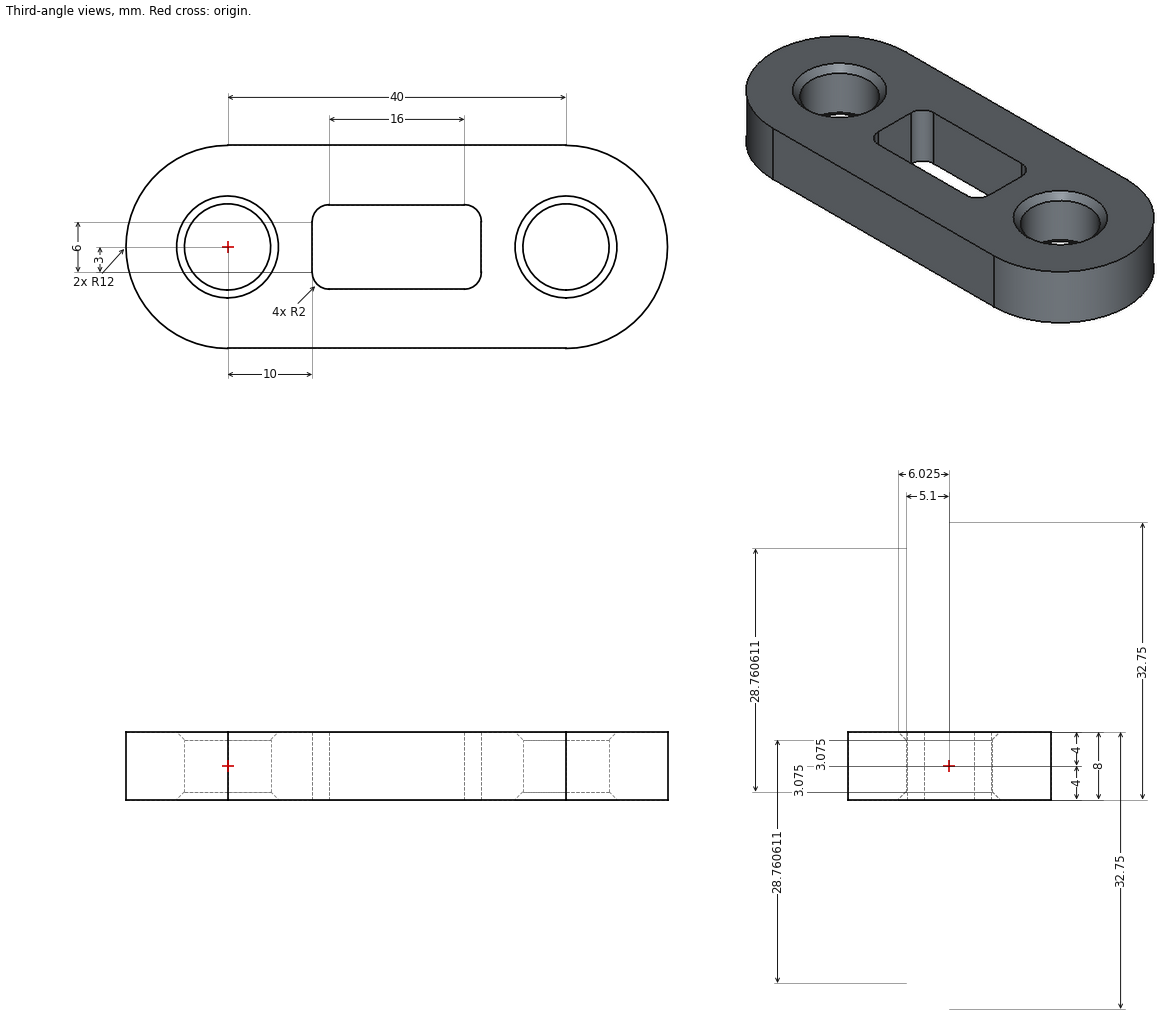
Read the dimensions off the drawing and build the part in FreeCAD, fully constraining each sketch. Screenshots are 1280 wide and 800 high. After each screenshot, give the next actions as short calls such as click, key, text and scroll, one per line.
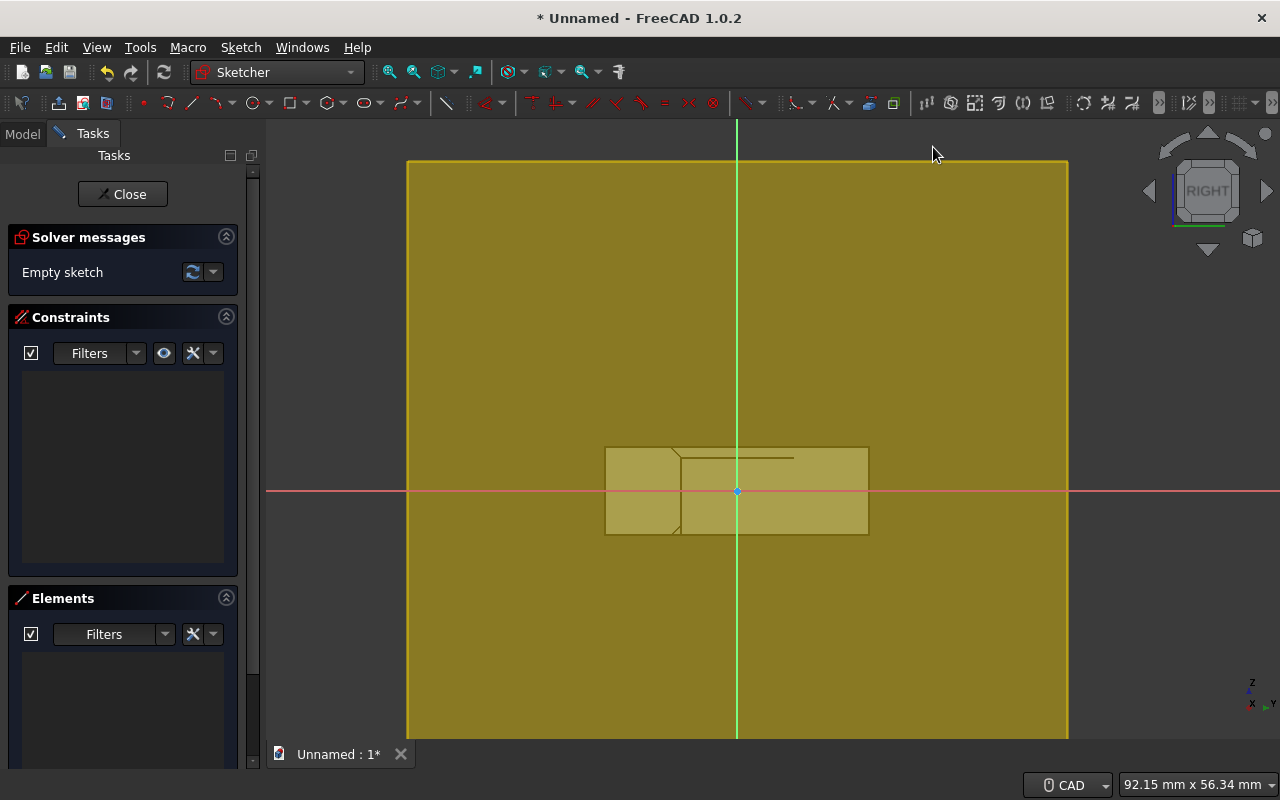
key(g)
key(m)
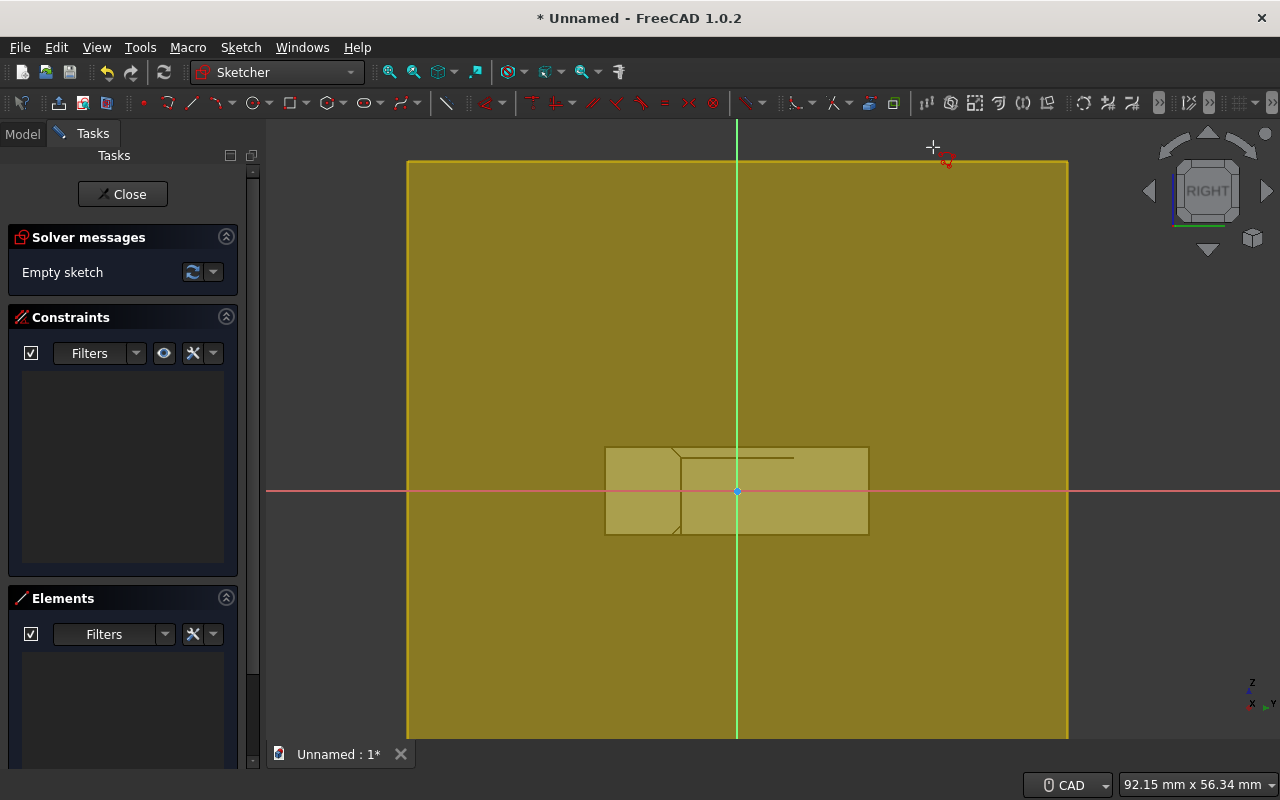
click(737, 535)
click(671, 535)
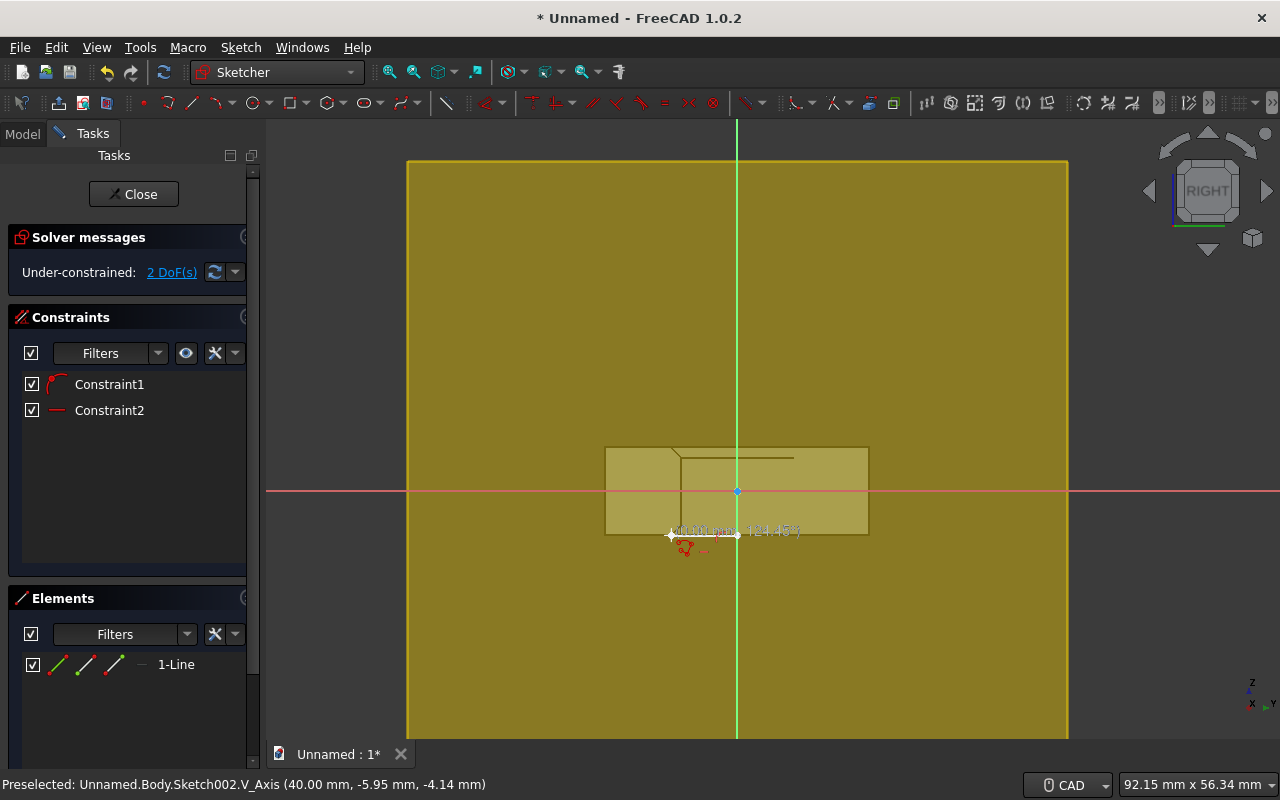
scroll(681, 525, up, 3)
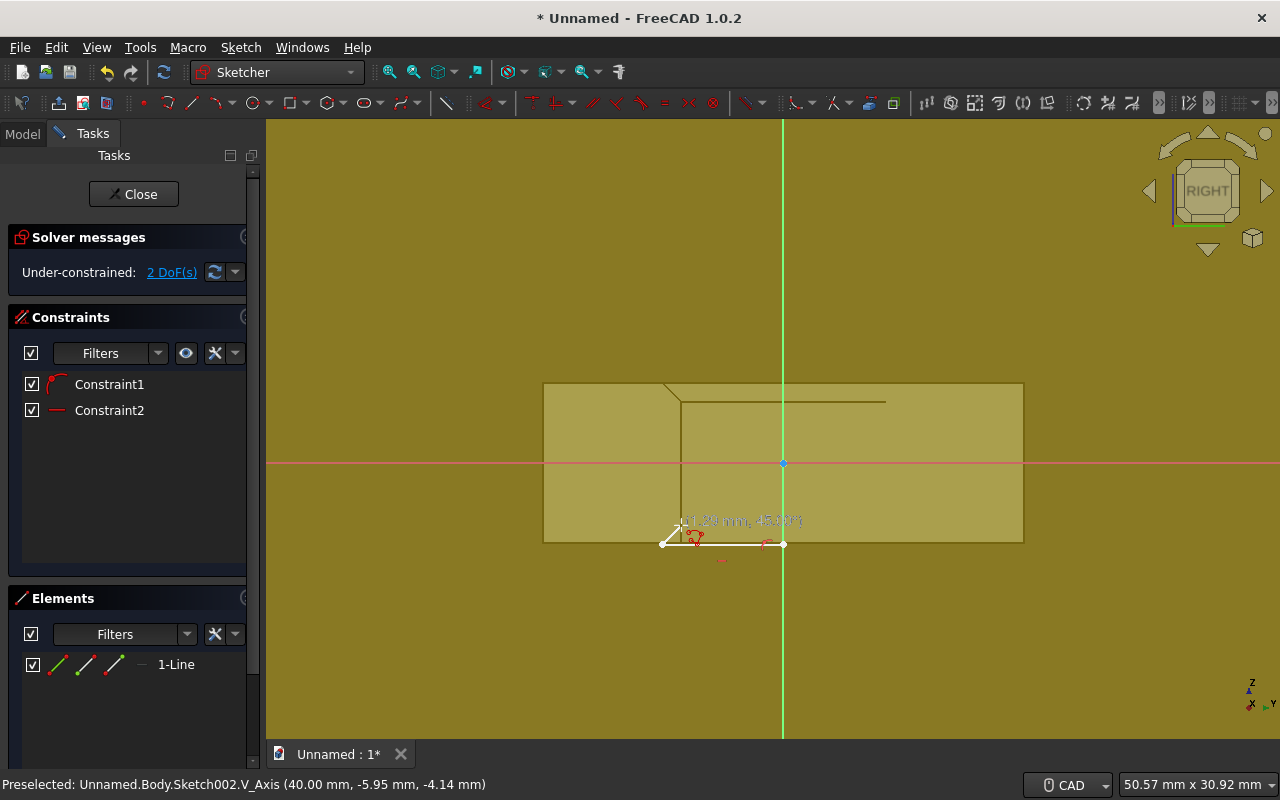
click(681, 525)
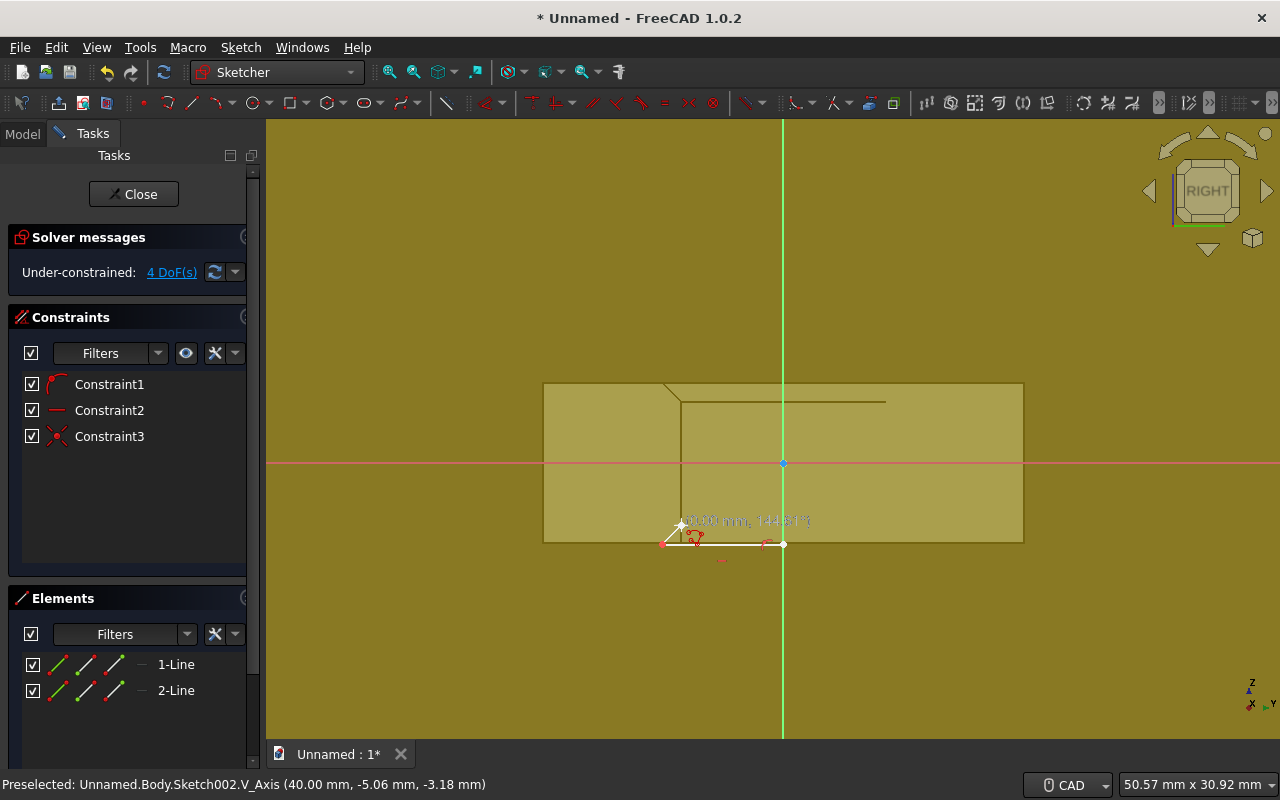
scroll(682, 689, down, 3)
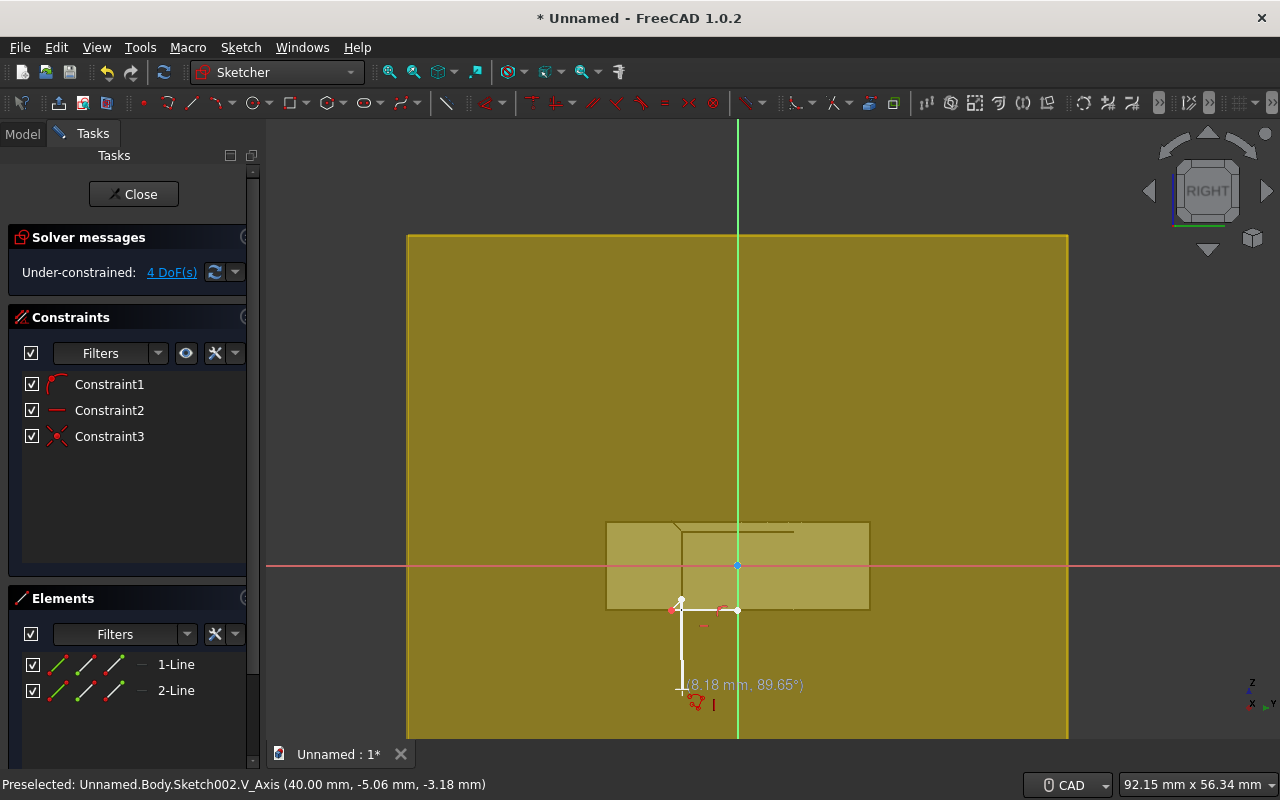
click(682, 283)
click(729, 249)
click(738, 610)
key(Escape)
key(Escape)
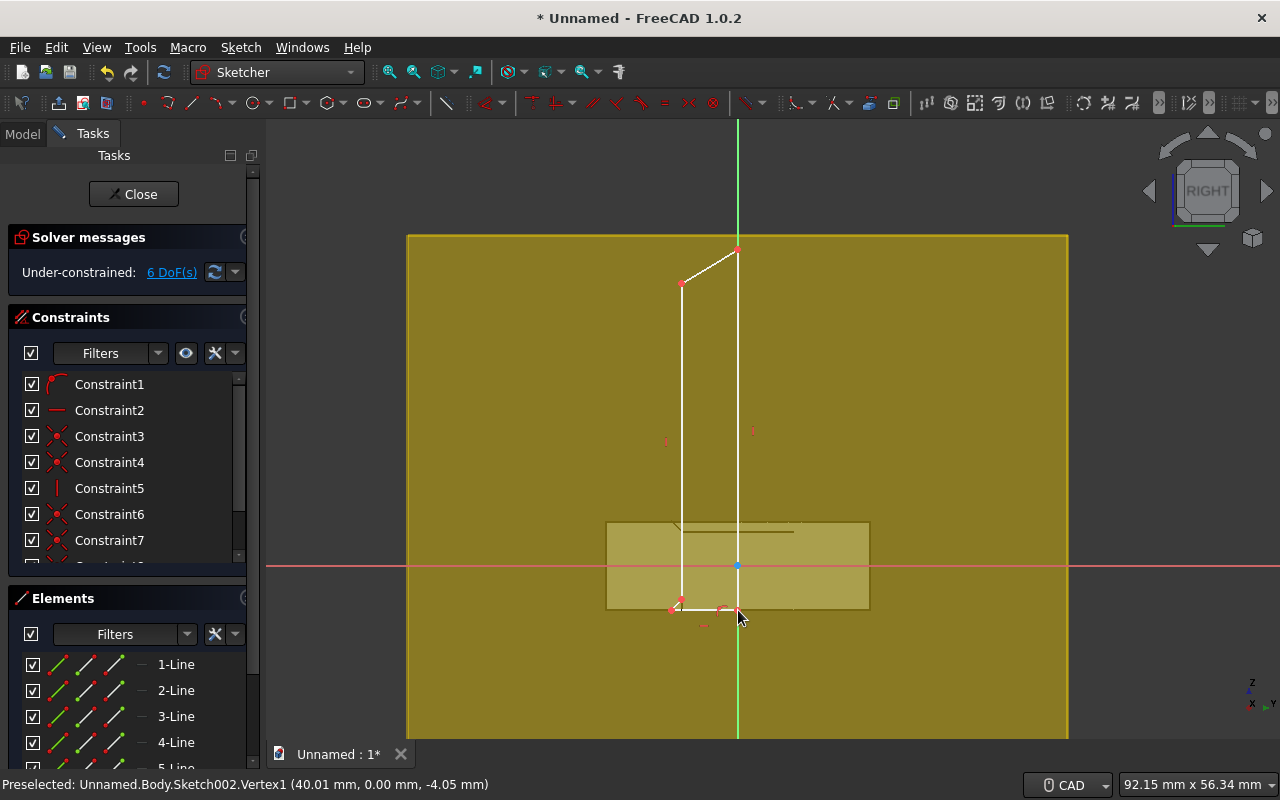
key(d)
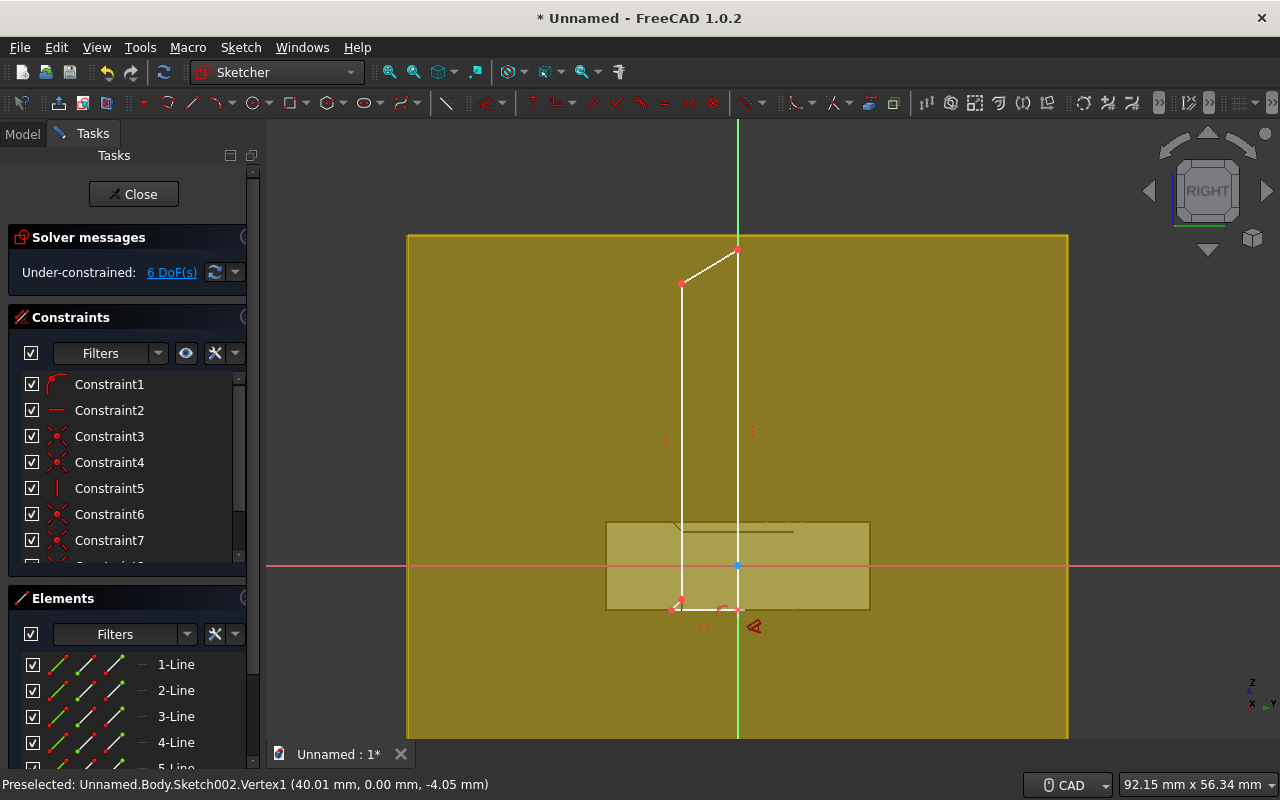
click(738, 610)
click(772, 588)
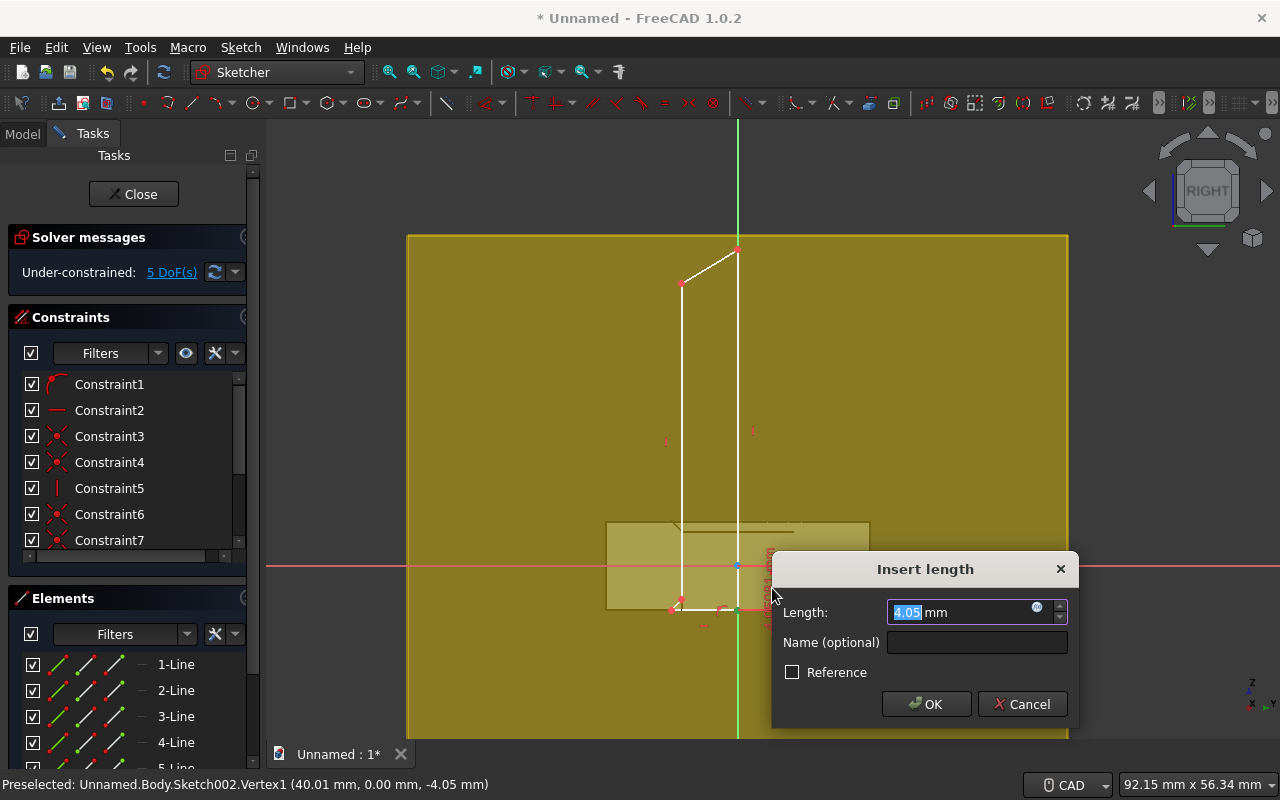
text(4)
key(Return)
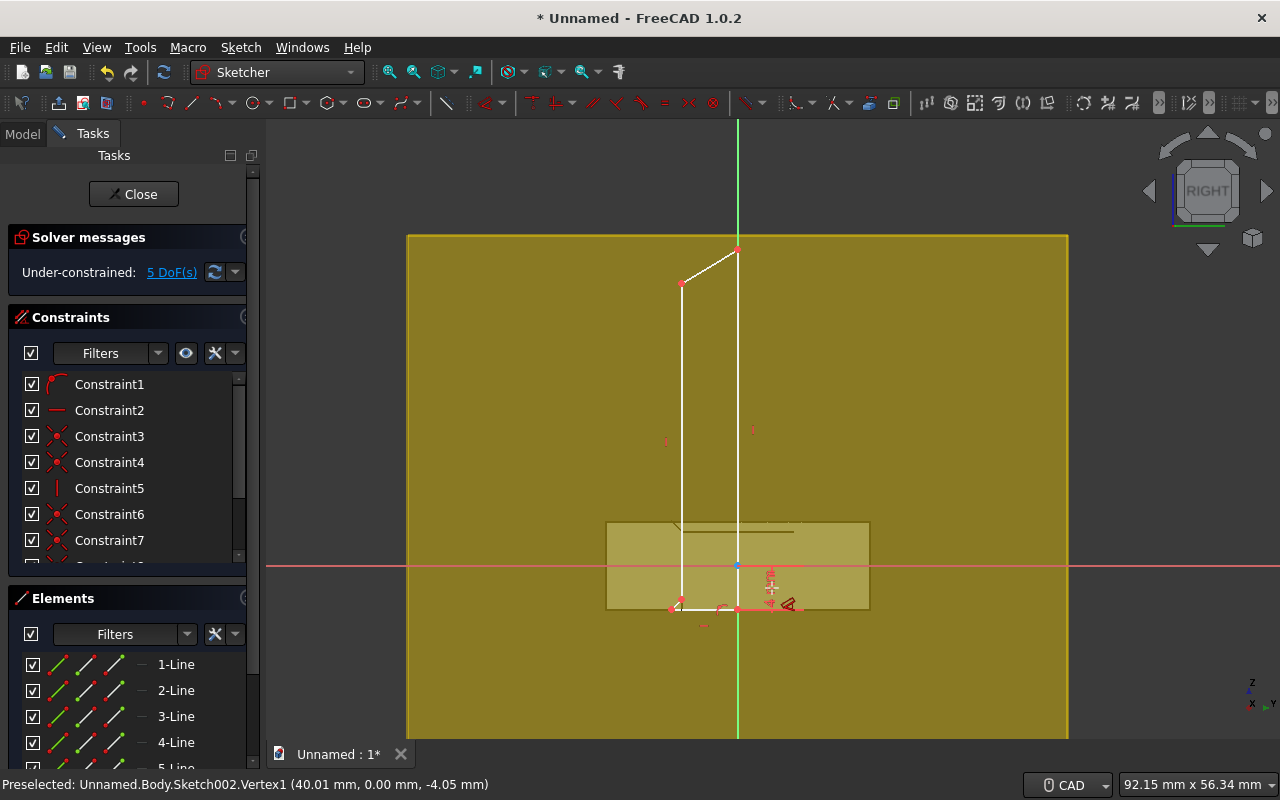
click(682, 600)
click(710, 634)